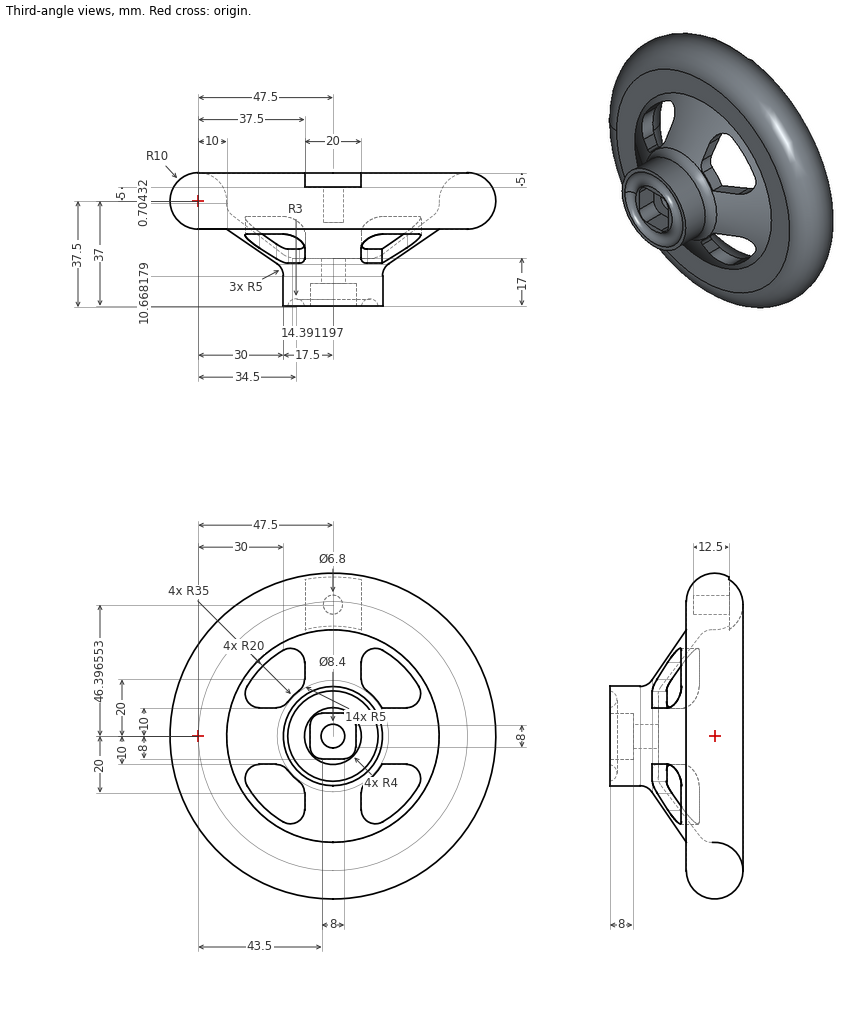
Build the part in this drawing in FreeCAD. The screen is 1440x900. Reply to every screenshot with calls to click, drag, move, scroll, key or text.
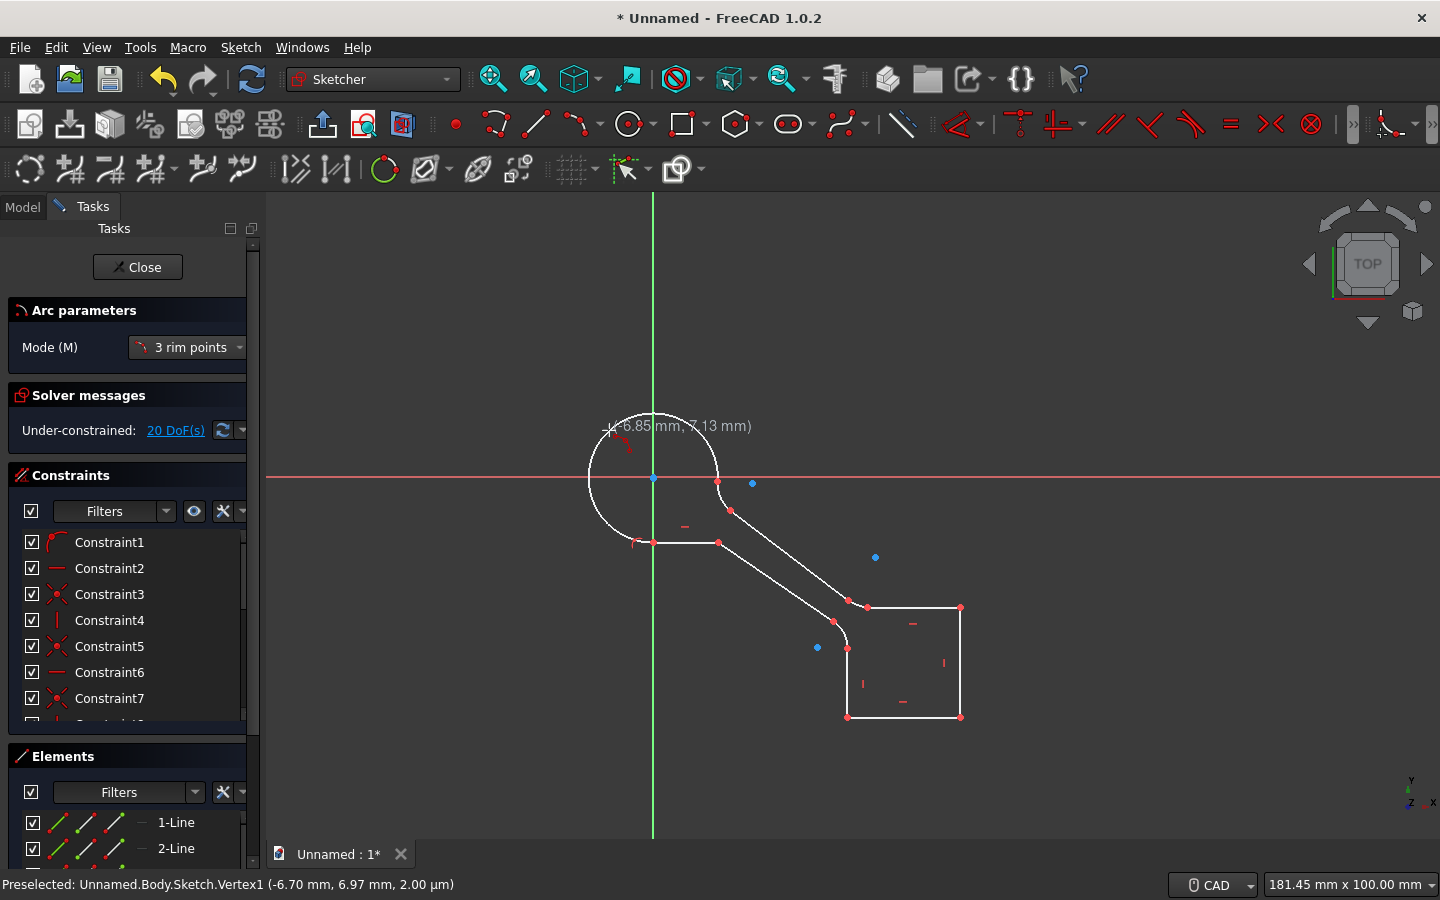
click(536, 124)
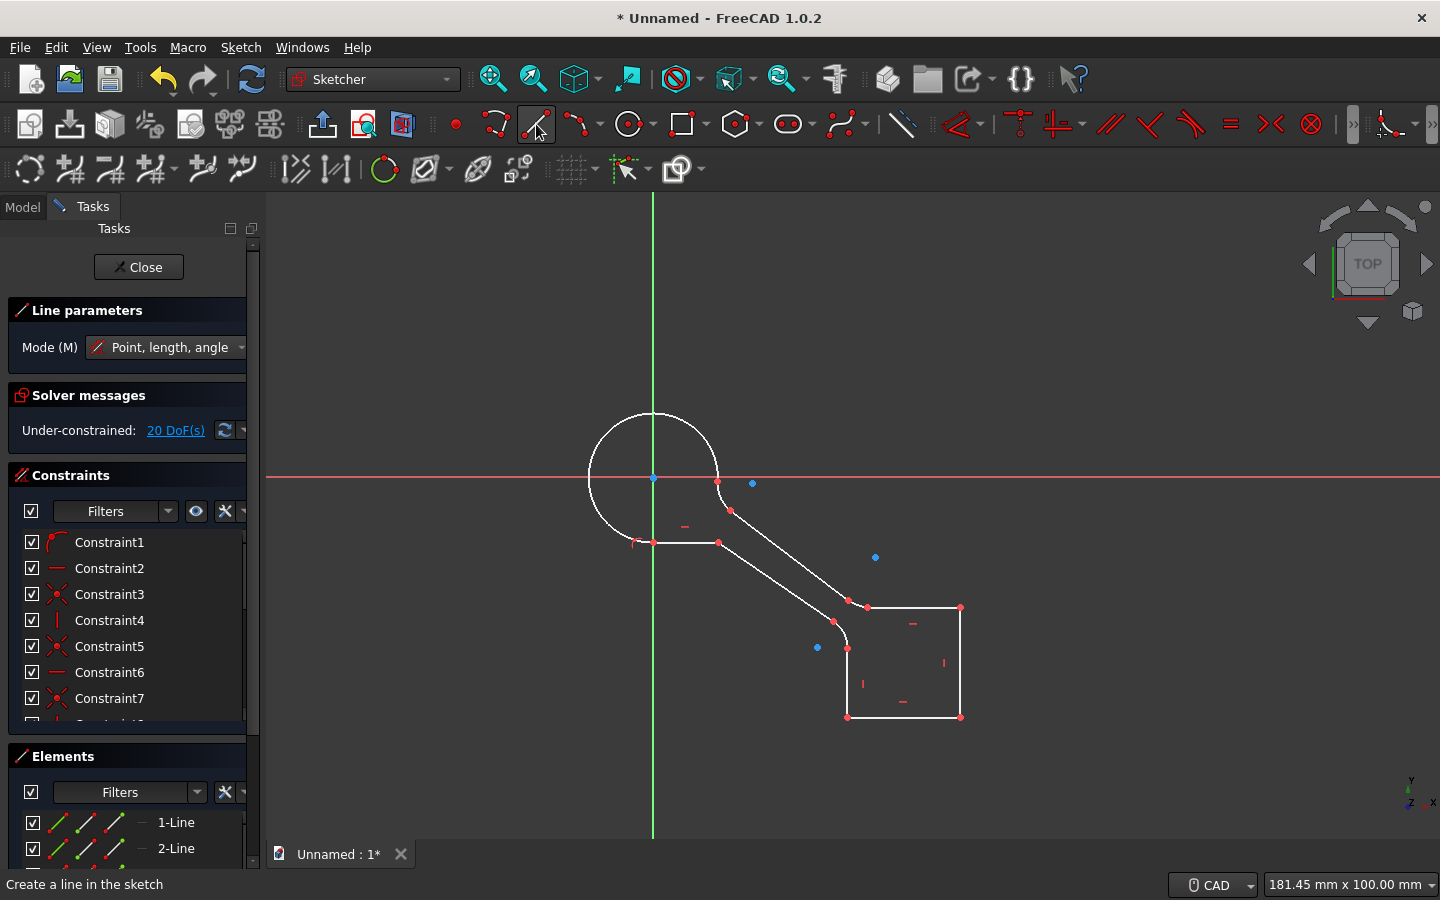
click(961, 401)
click(961, 315)
key(Escape)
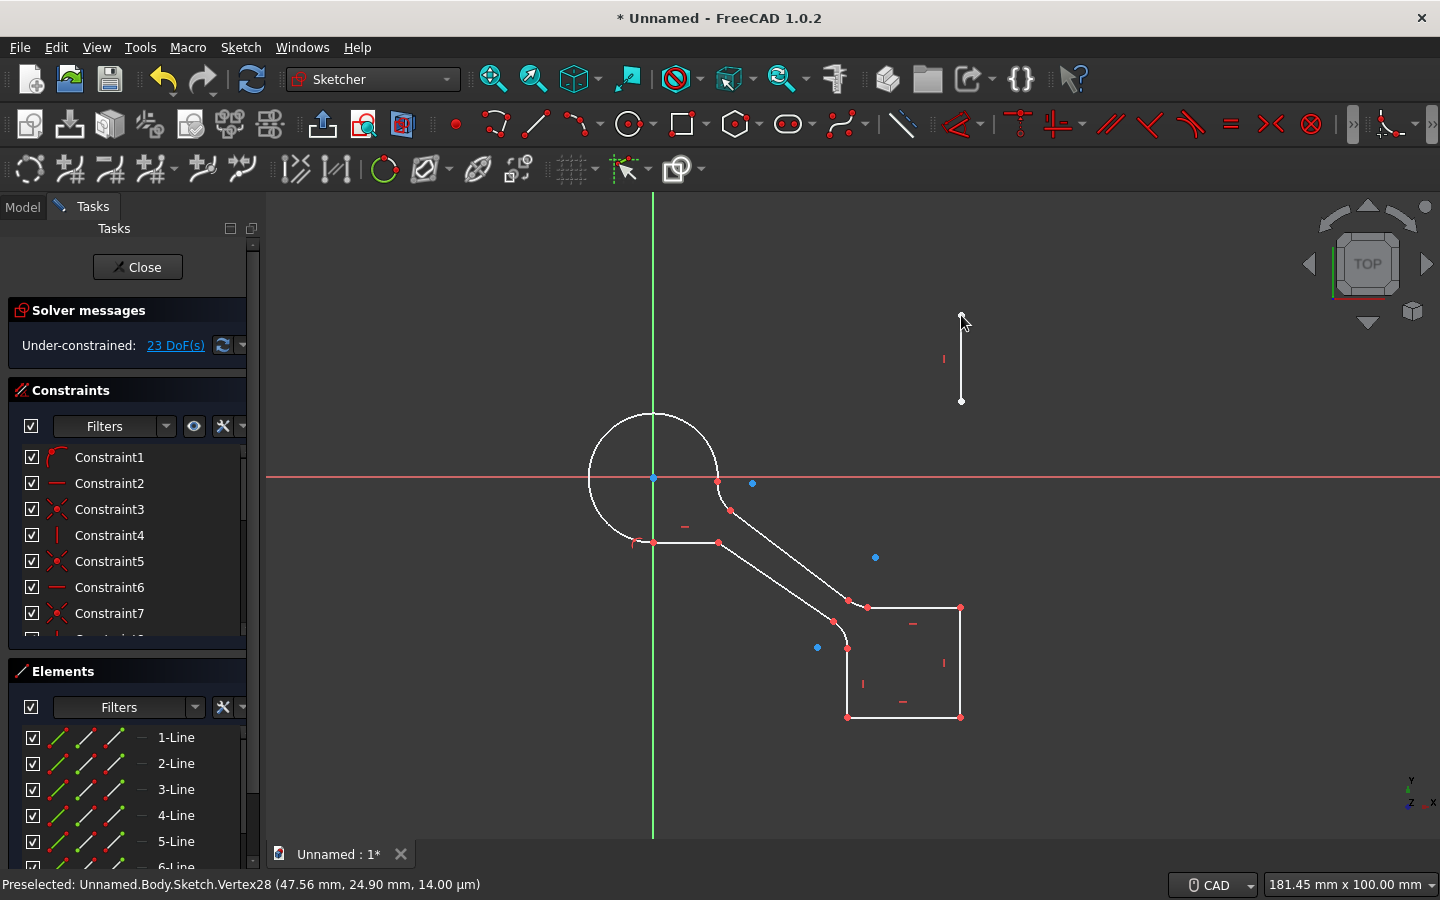
click(961, 376)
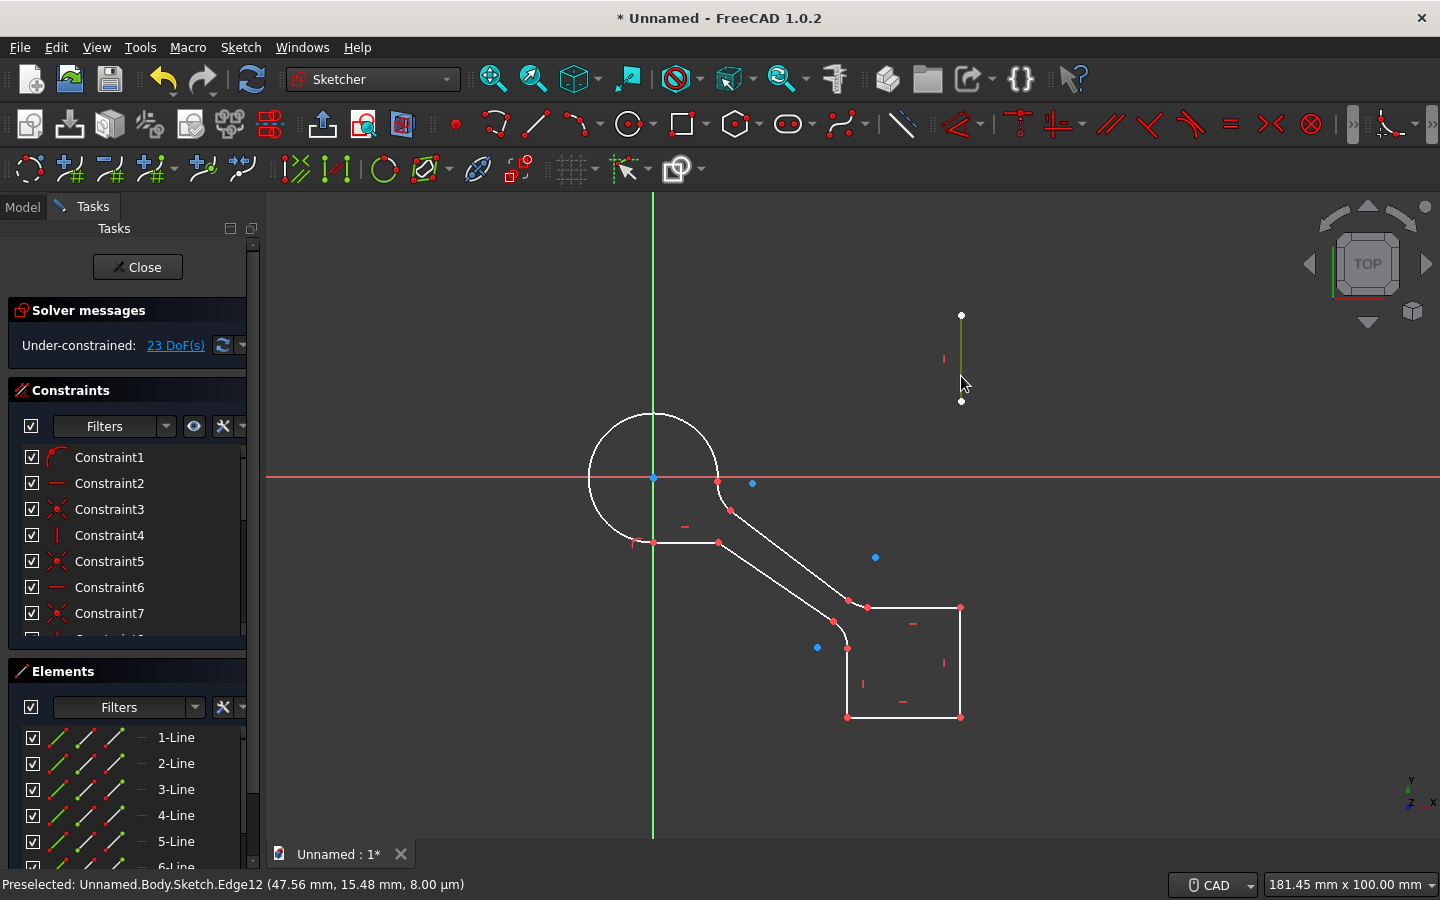
click(904, 124)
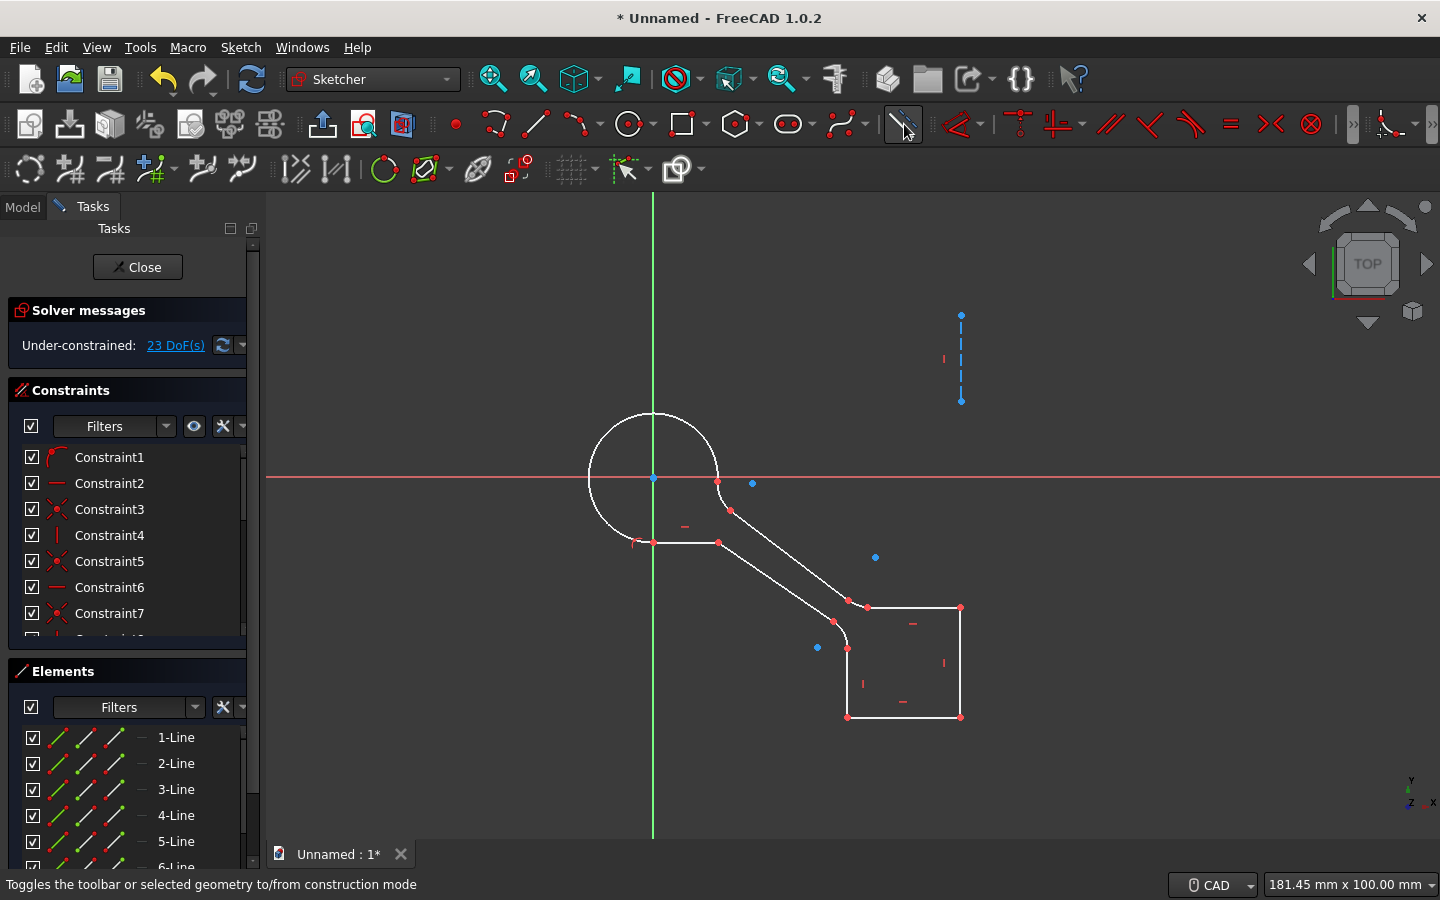
click(673, 543)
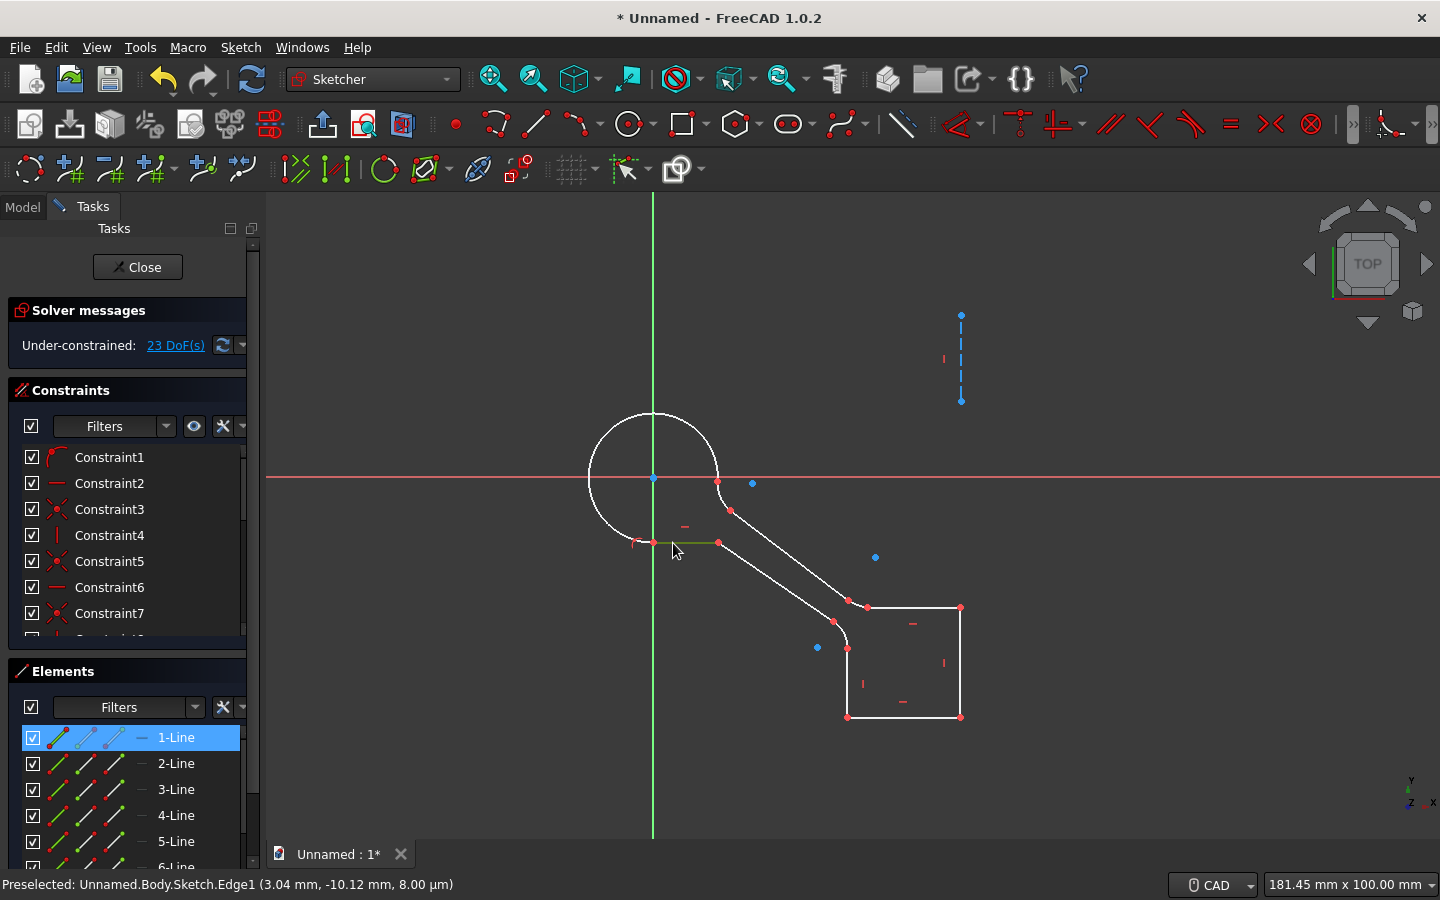
click(666, 415)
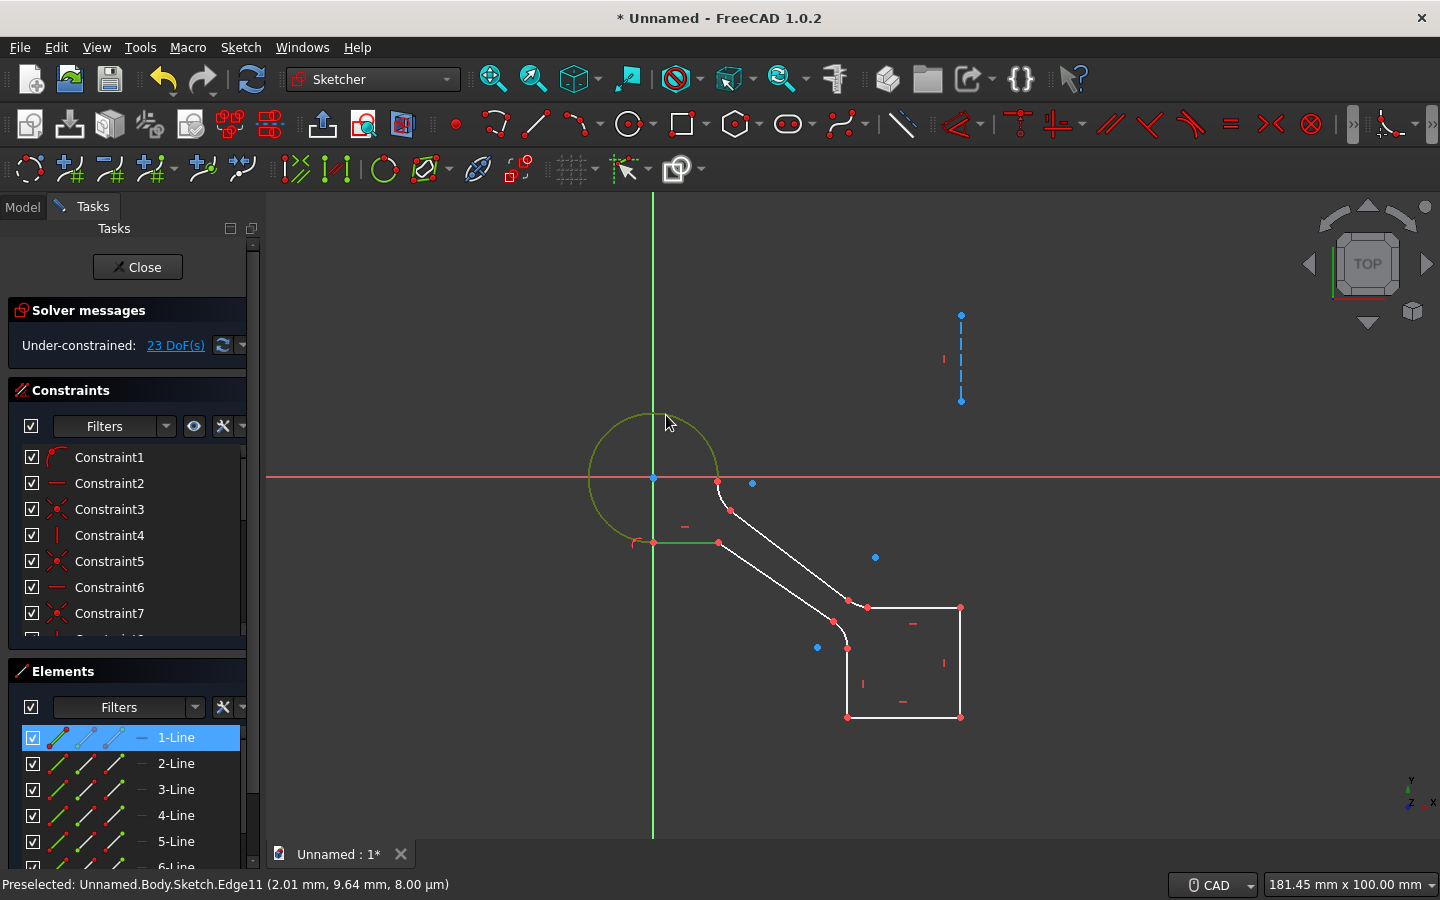
click(1192, 124)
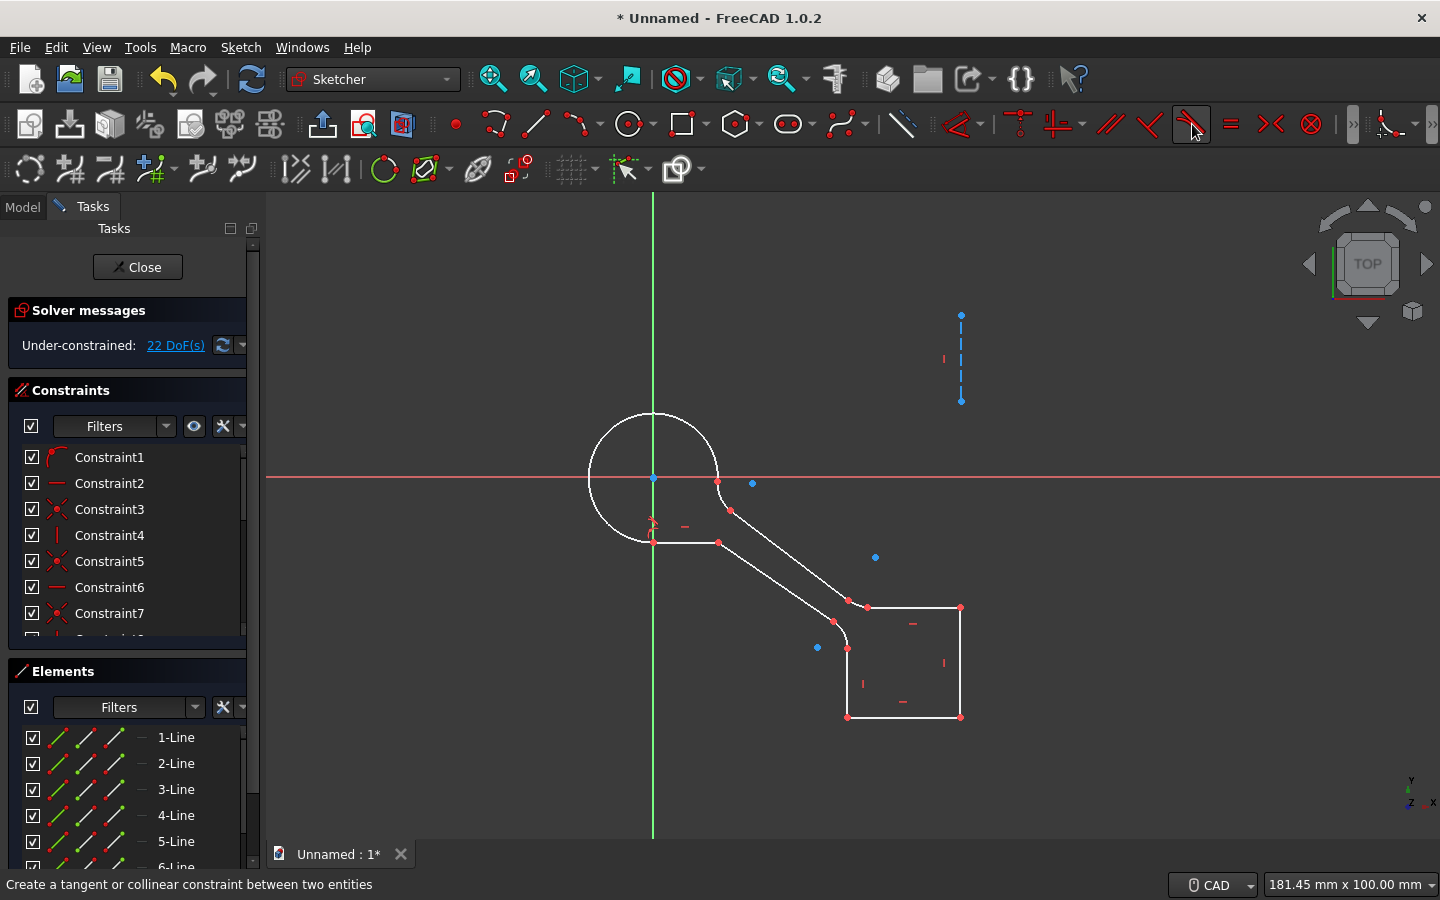
click(753, 566)